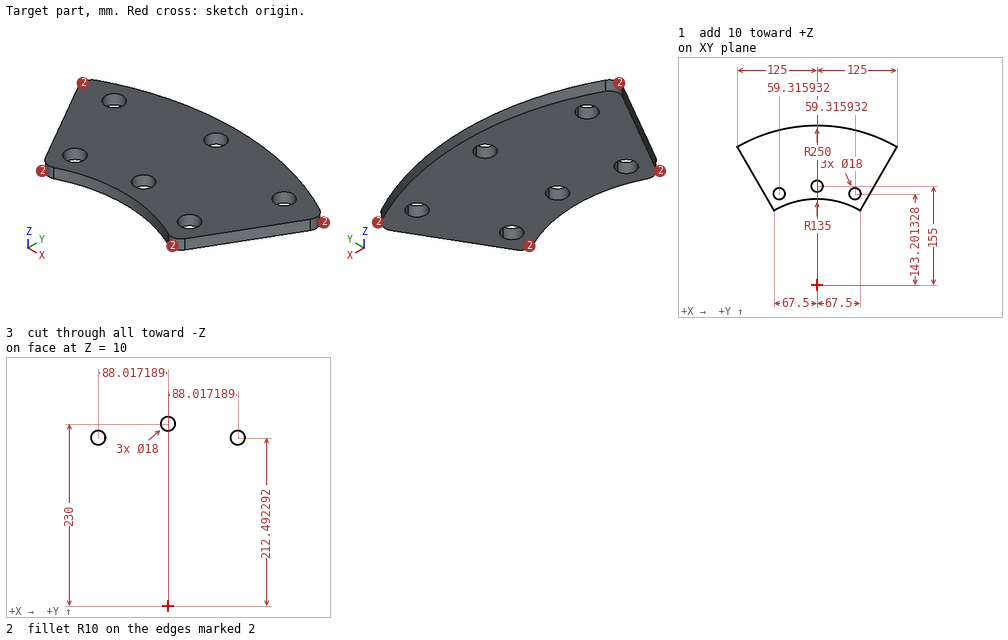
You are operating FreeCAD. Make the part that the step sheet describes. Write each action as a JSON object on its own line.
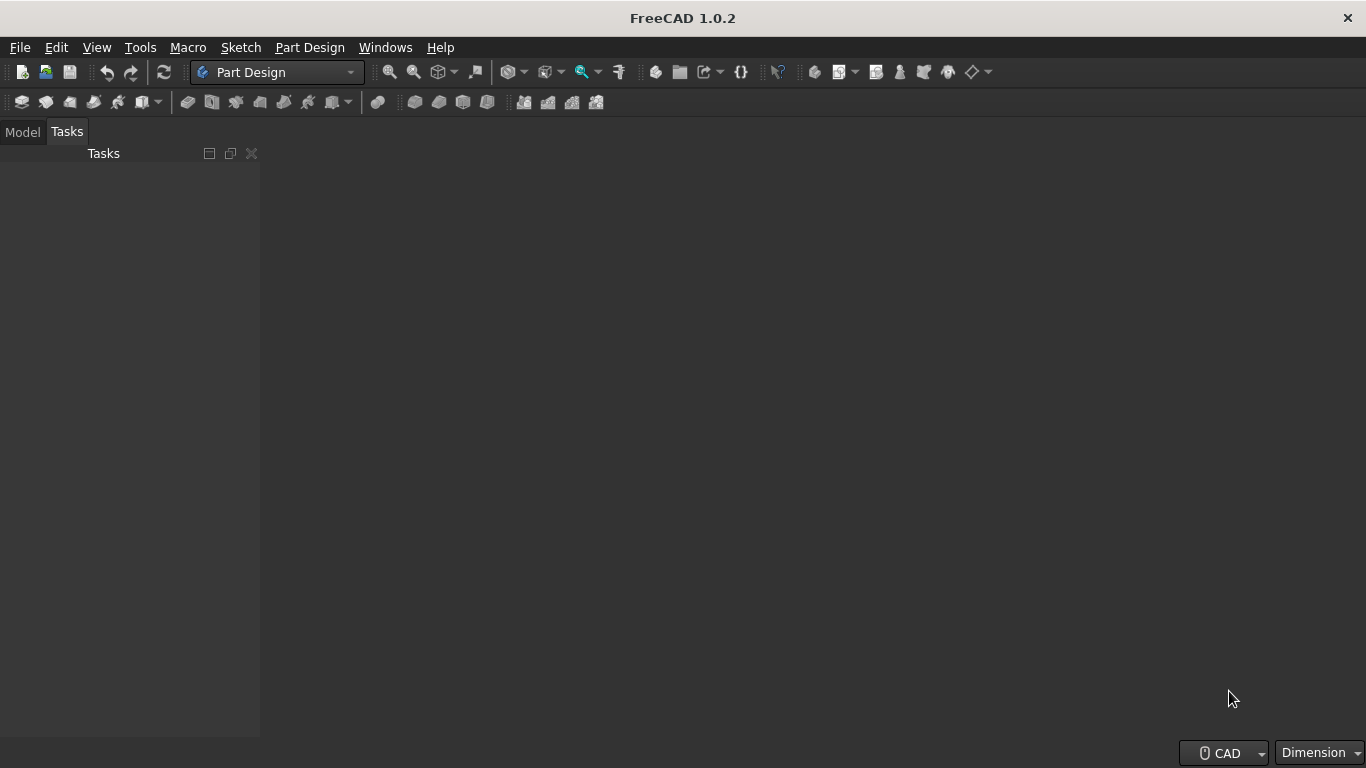
{"action": "left_click", "coordinate": [22, 72]}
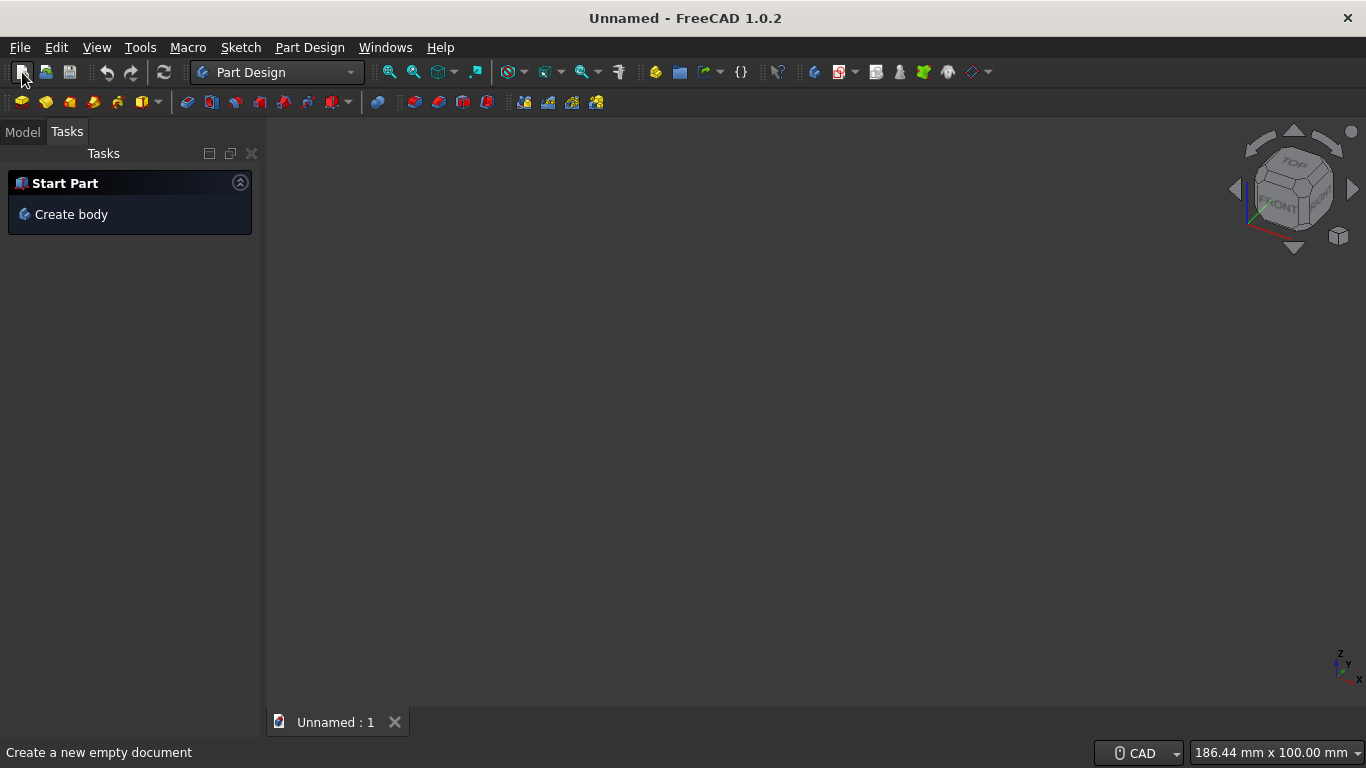
{"action": "left_click", "coordinate": [840, 72]}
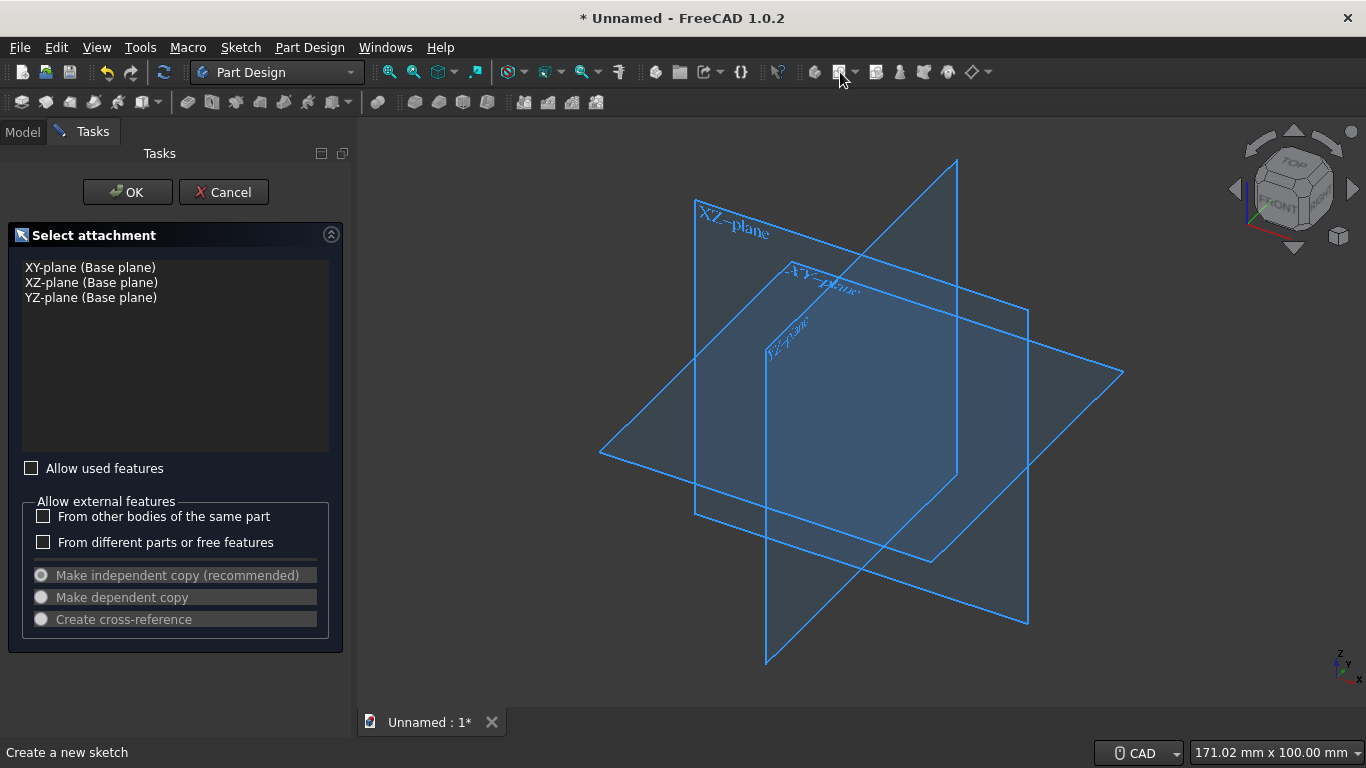
{"action": "left_click", "coordinate": [82, 268]}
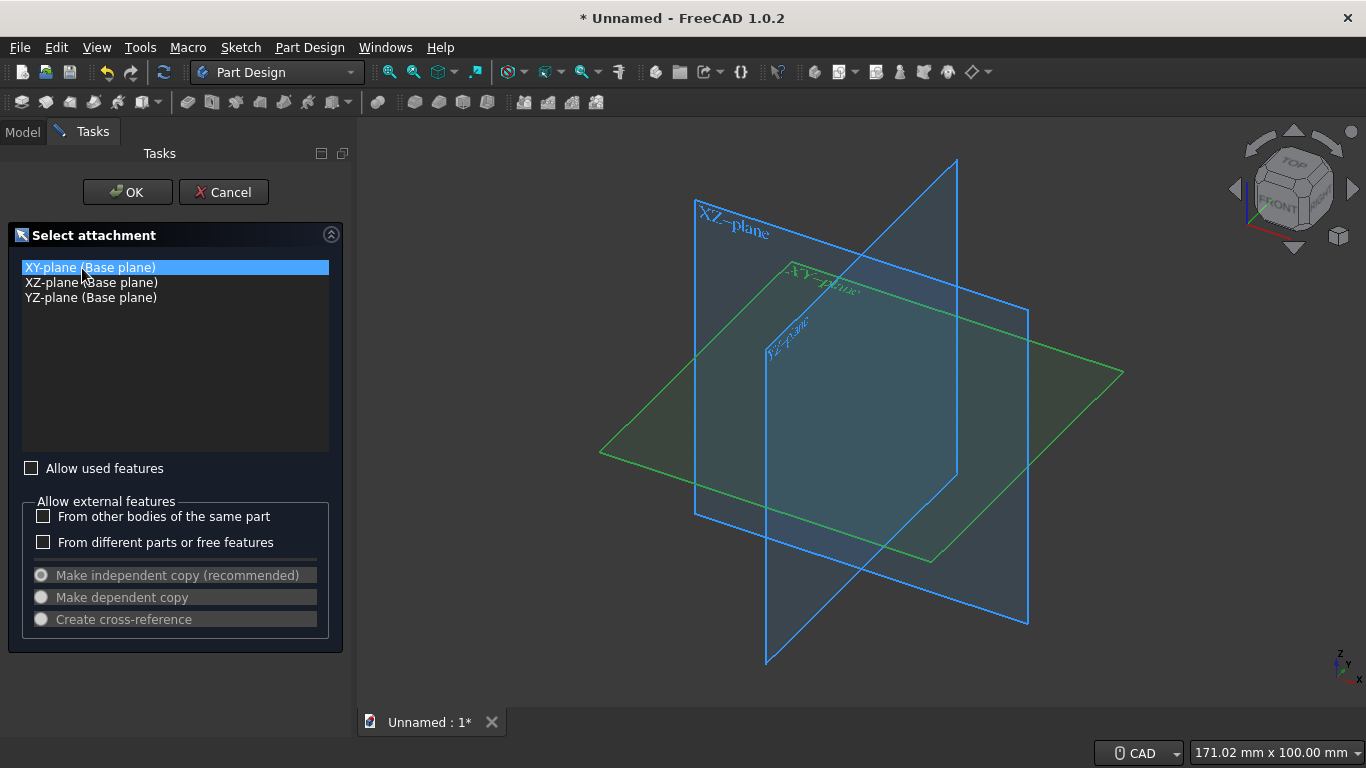
{"action": "left_click", "coordinate": [128, 192]}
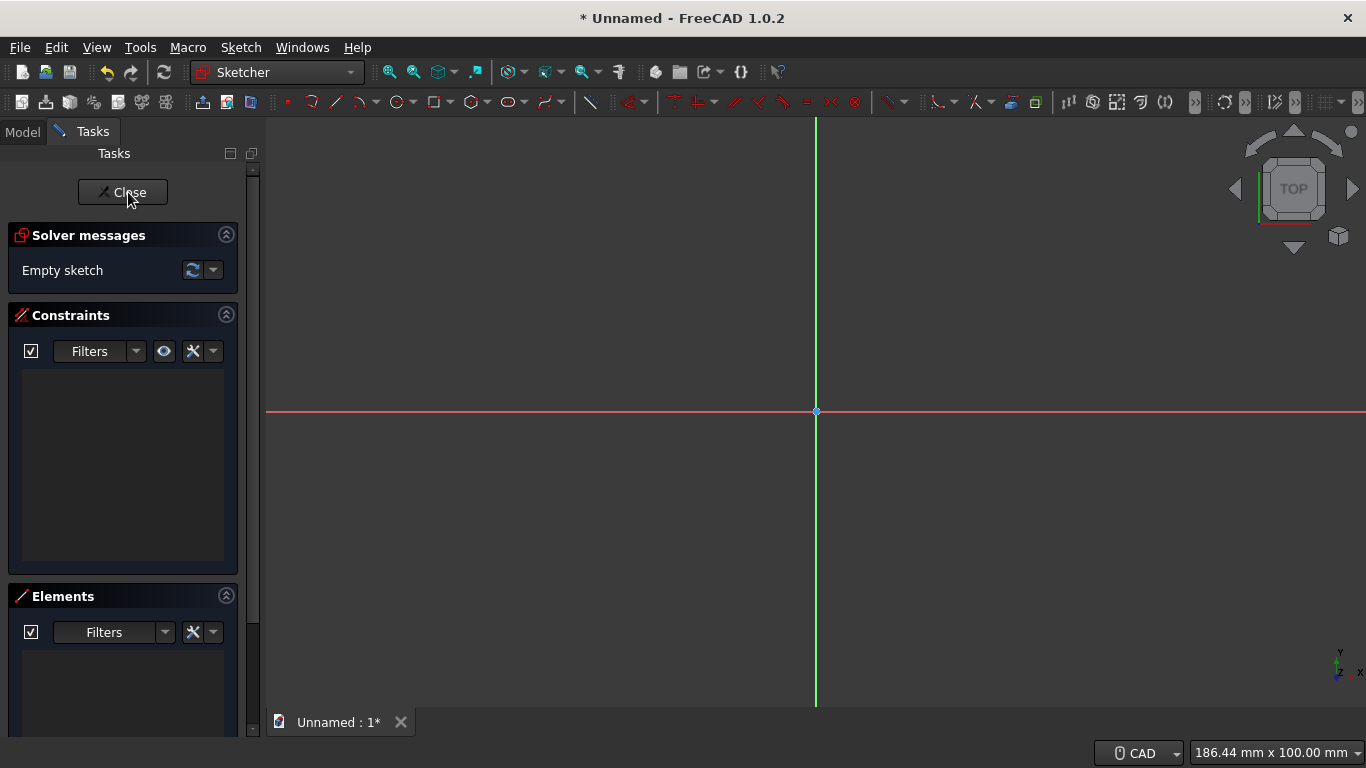
{"action": "scroll", "coordinate": [725, 653], "scroll_direction": "down", "scroll_amount": 7}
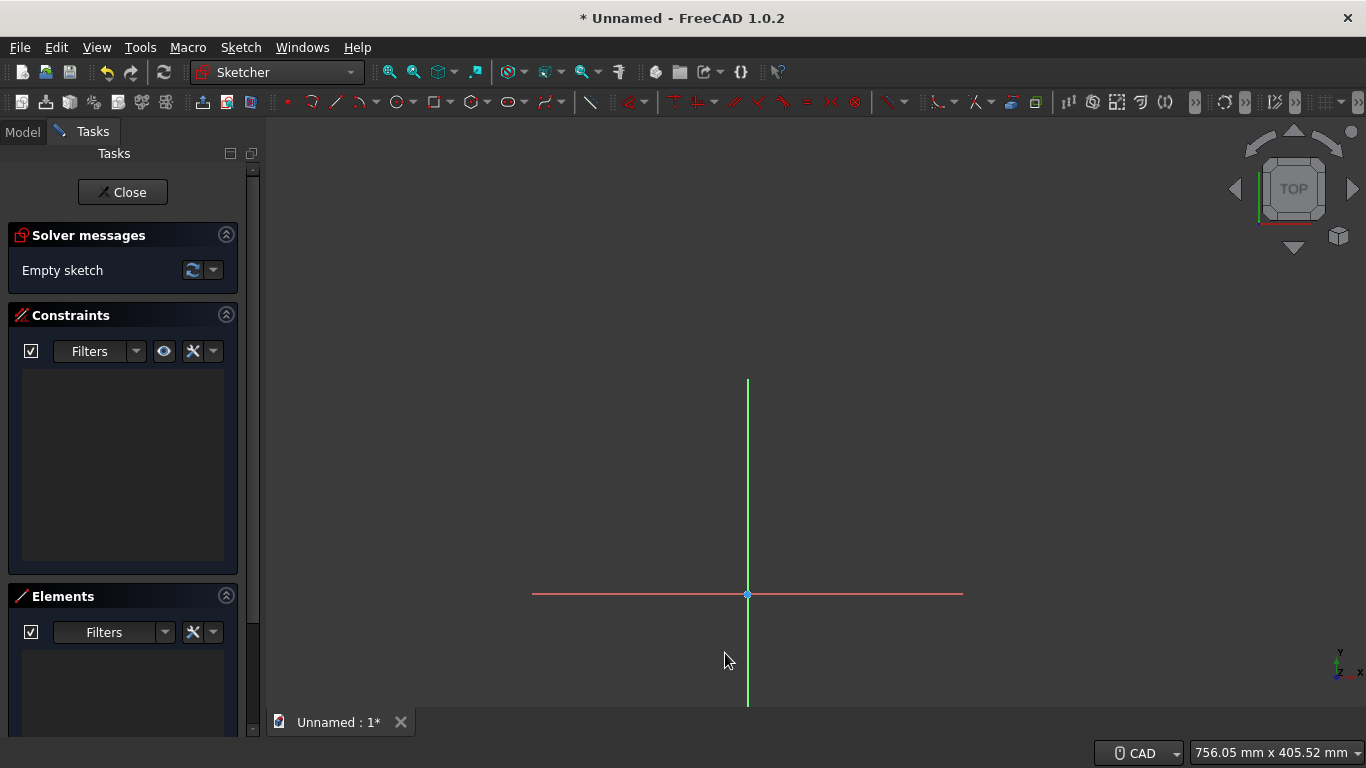
{"action": "left_click", "coordinate": [336, 102]}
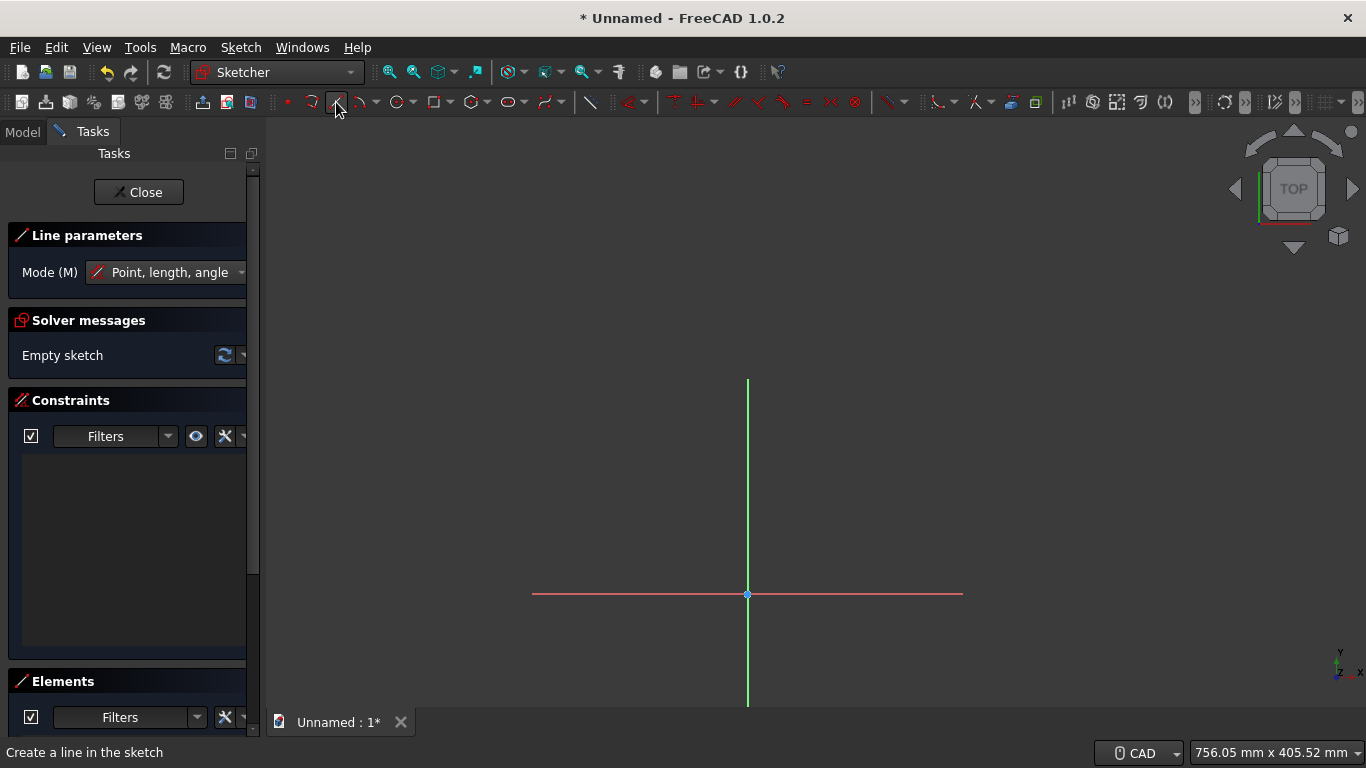
{"action": "left_click", "coordinate": [566, 279]}
{"action": "left_click", "coordinate": [650, 424]}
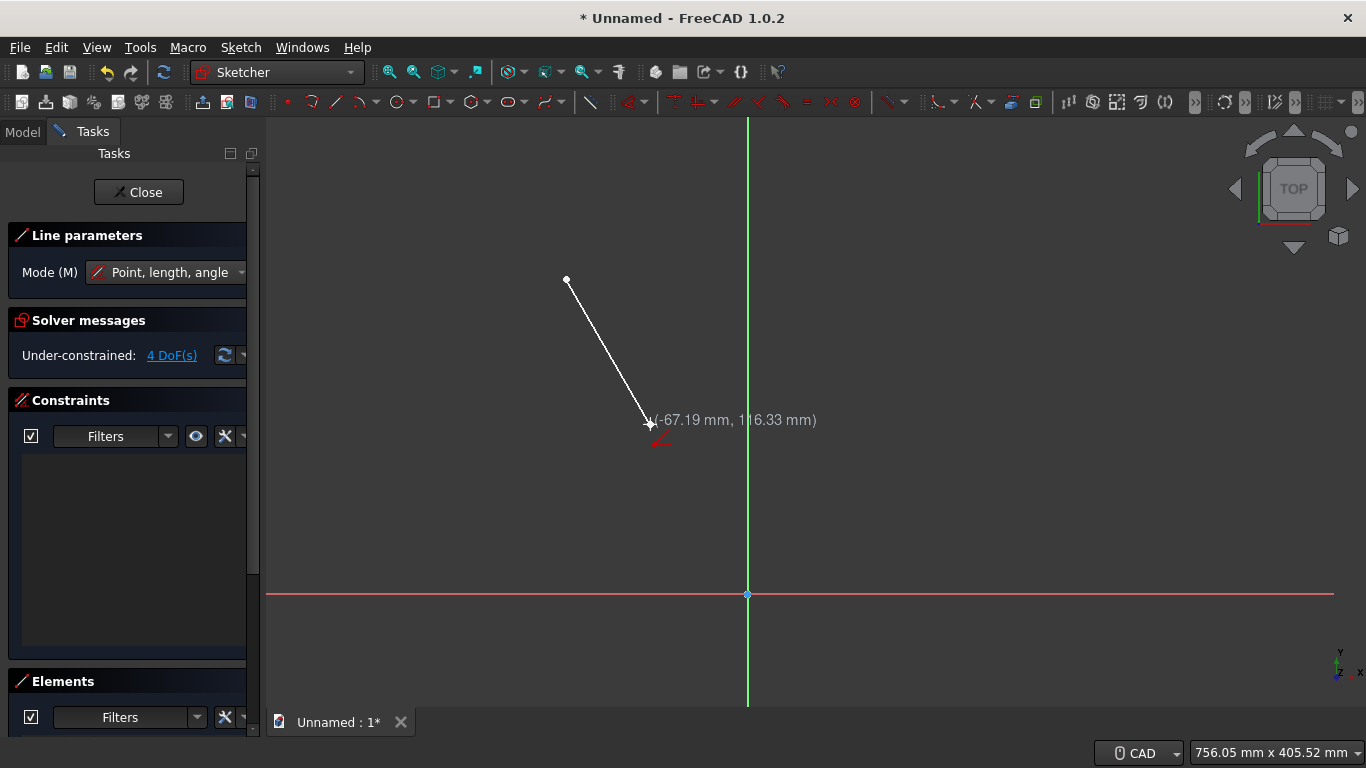
{"action": "left_click", "coordinate": [846, 424]}
{"action": "left_click", "coordinate": [930, 279]}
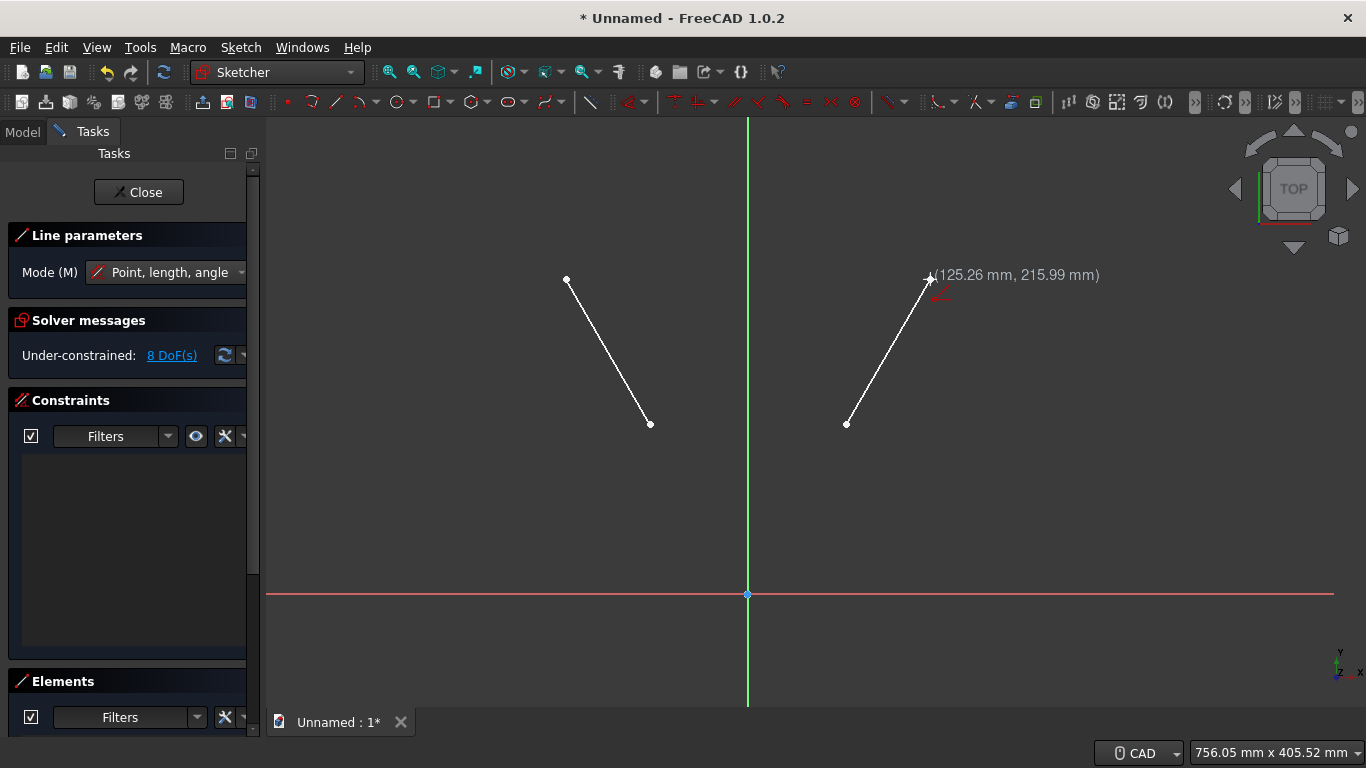
{"action": "key", "text": "g 3 a"}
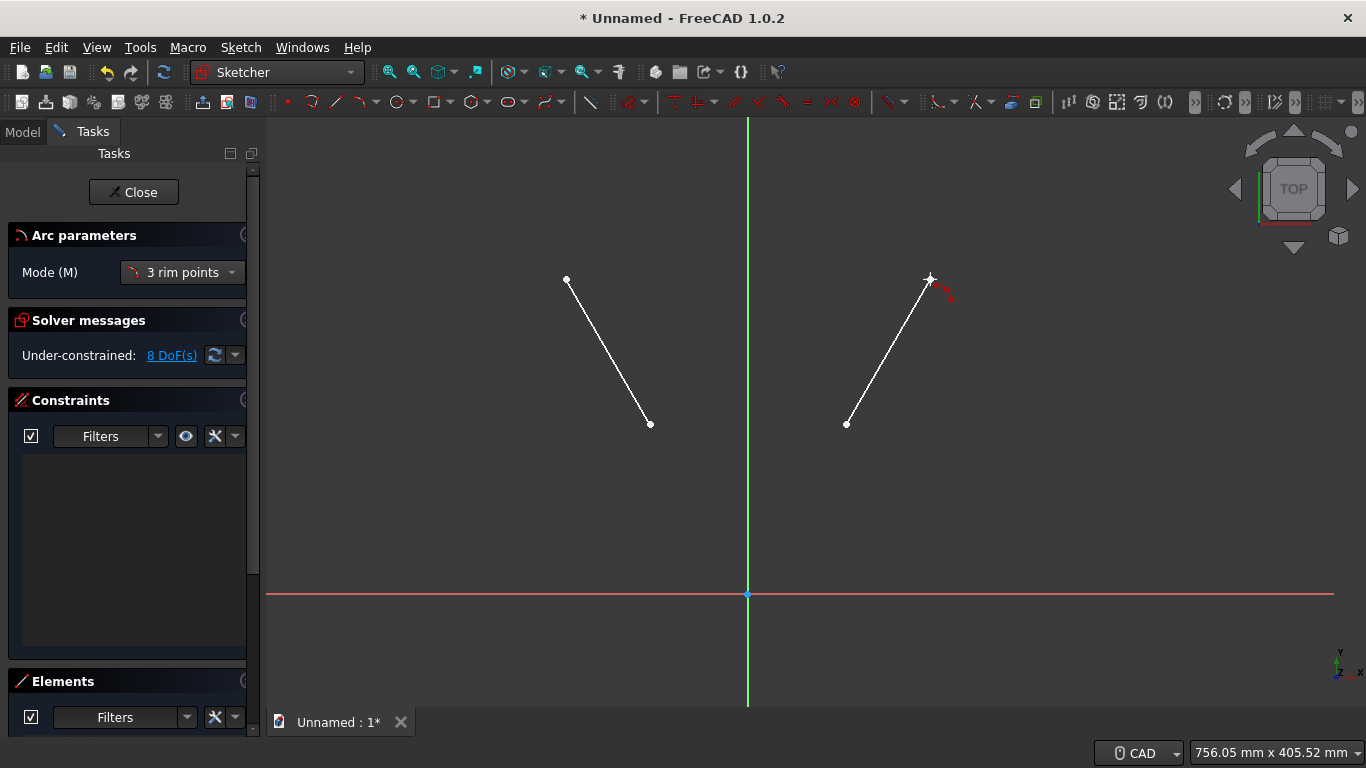
{"action": "left_click", "coordinate": [650, 425]}
{"action": "left_click", "coordinate": [846, 425]}
{"action": "left_click", "coordinate": [768, 399]}